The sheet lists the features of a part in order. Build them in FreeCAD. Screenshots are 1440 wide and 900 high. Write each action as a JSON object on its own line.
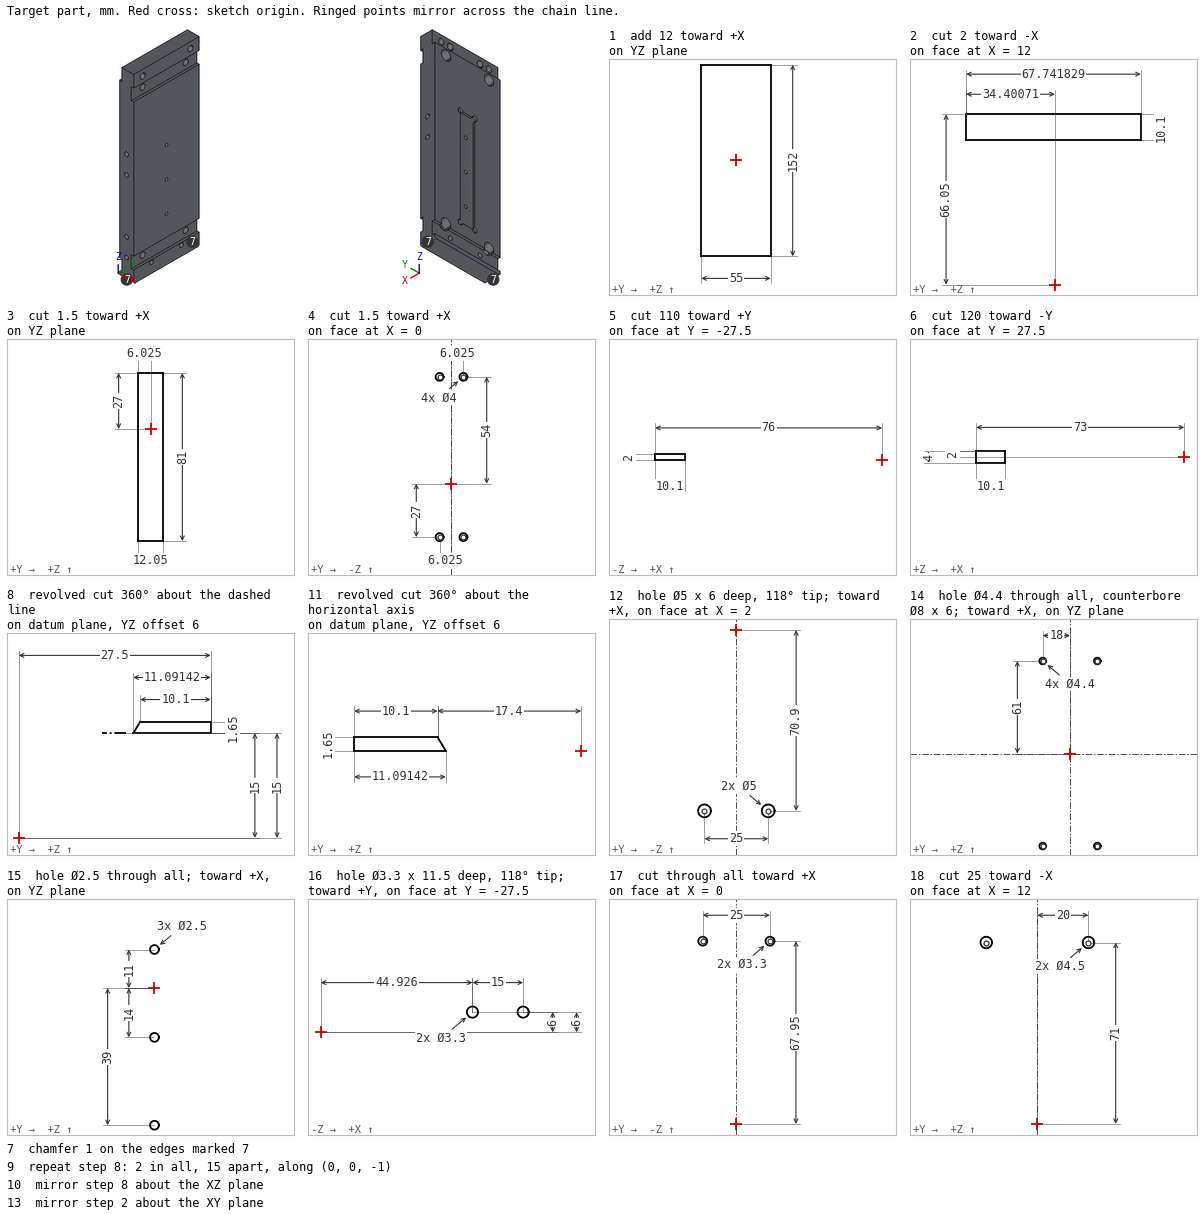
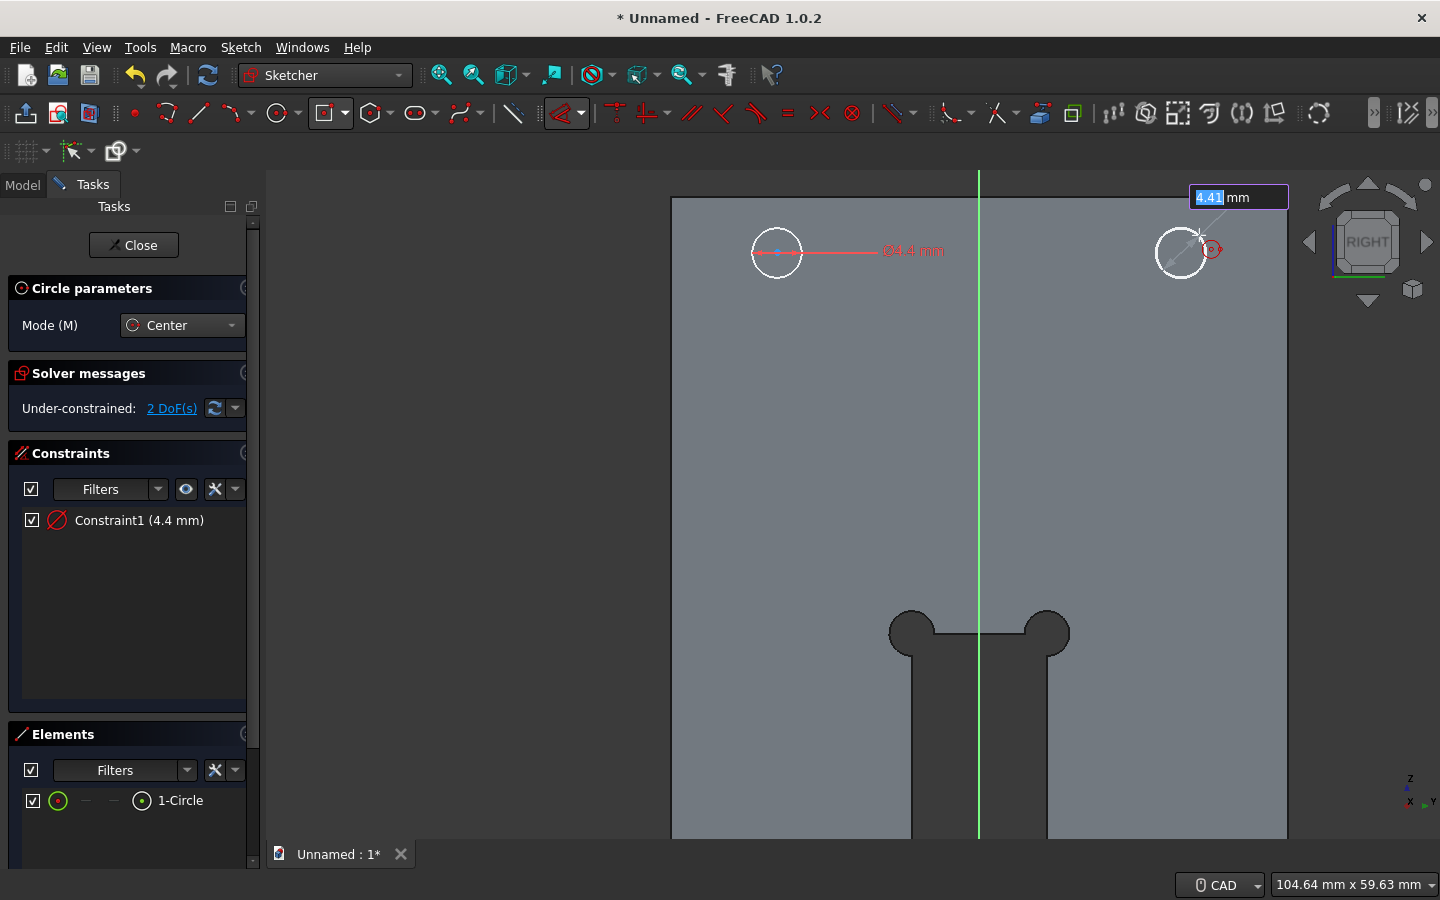
{"action": "type", "text": "4.4"}
{"action": "key", "text": "Return"}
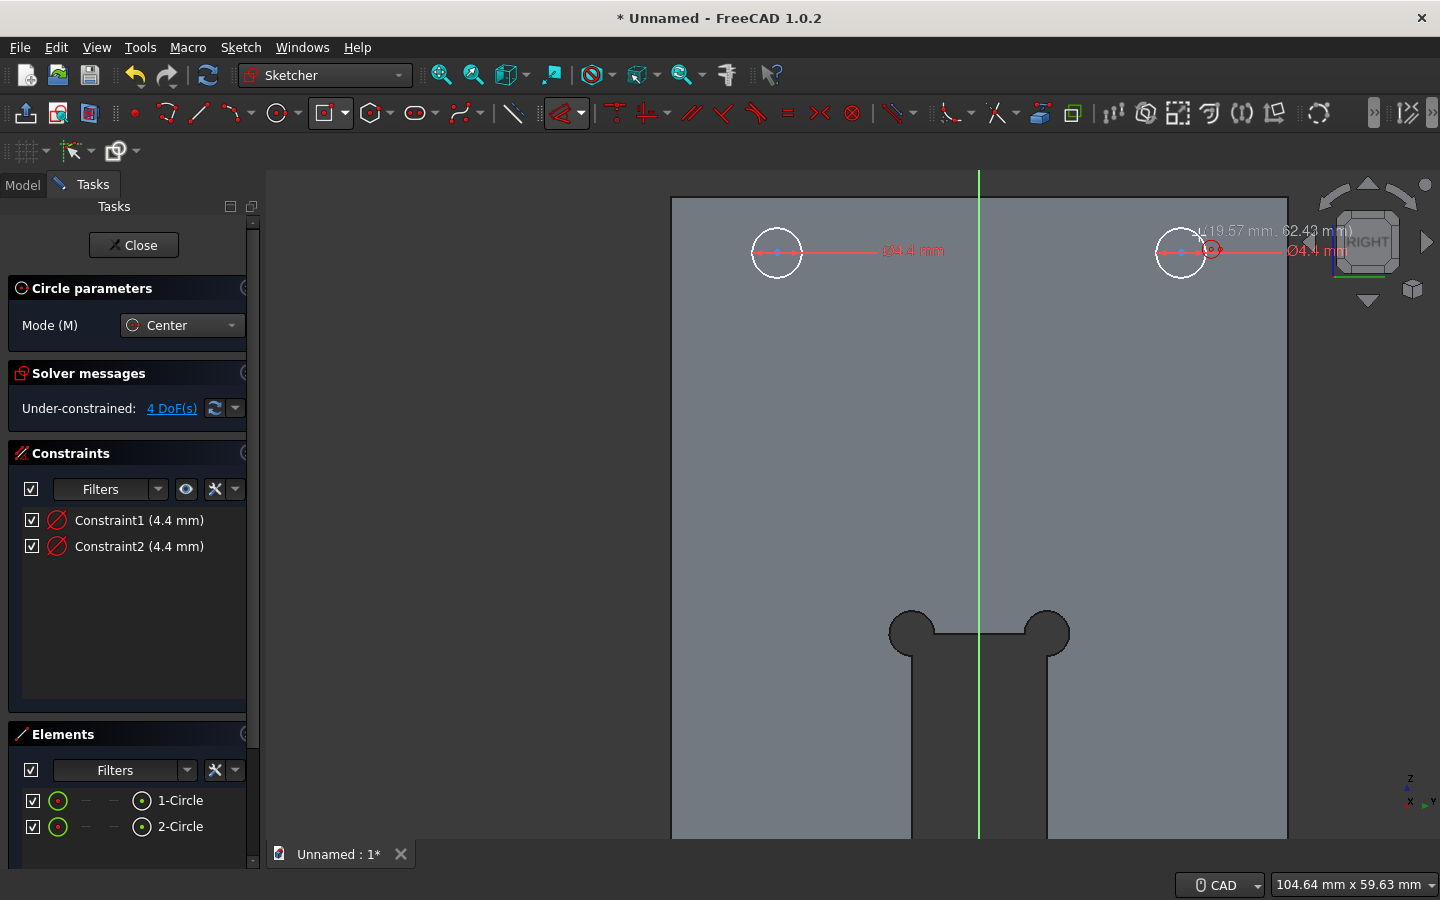
{"action": "scroll", "coordinate": [700, 318], "scroll_direction": "down", "scroll_amount": 6}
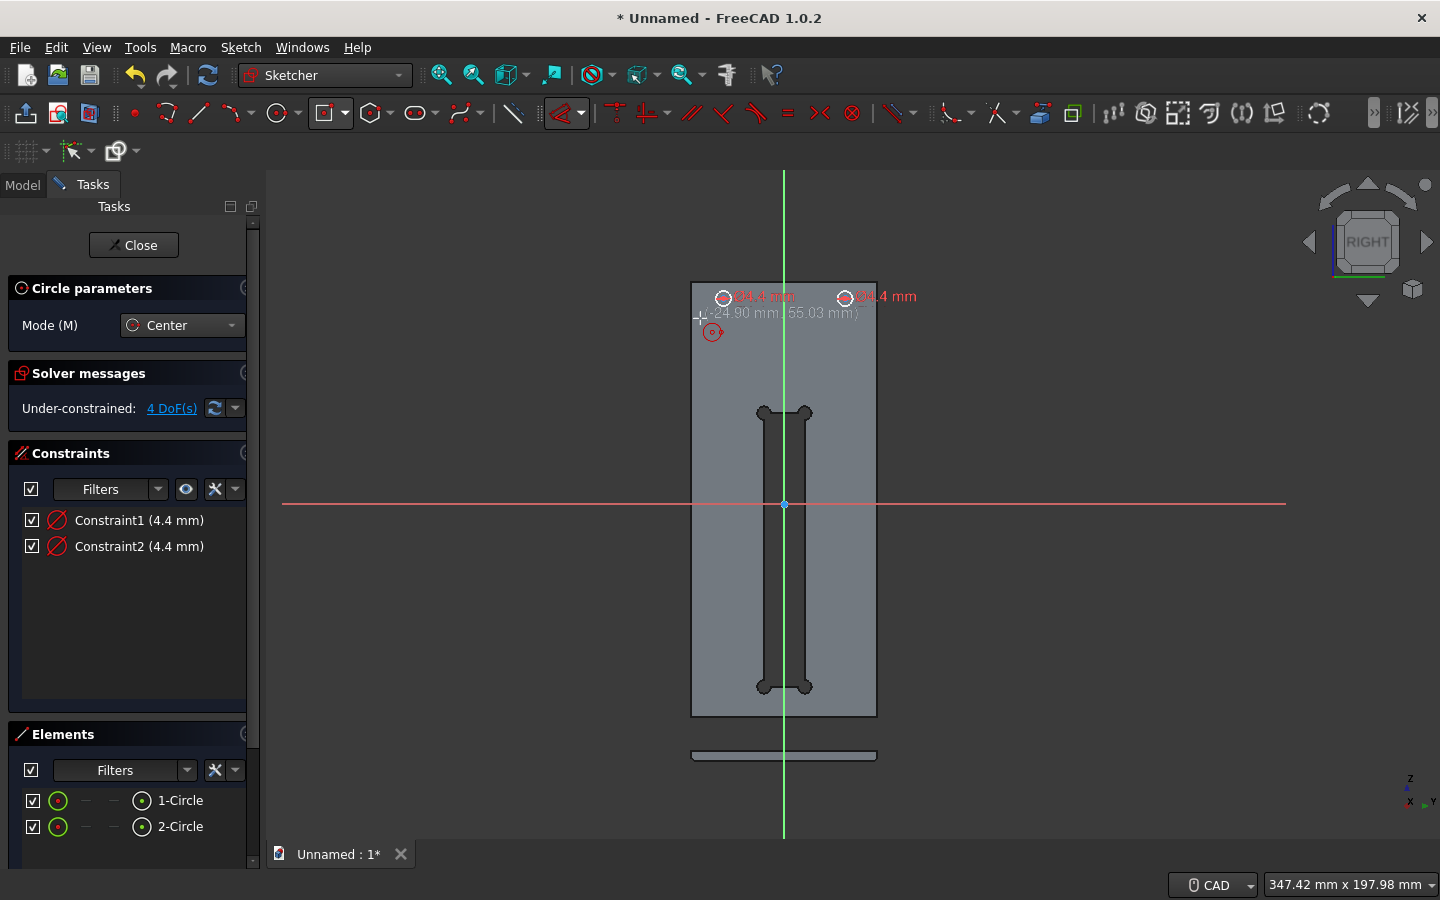
{"action": "scroll", "coordinate": [845, 711], "scroll_direction": "up", "scroll_amount": 6}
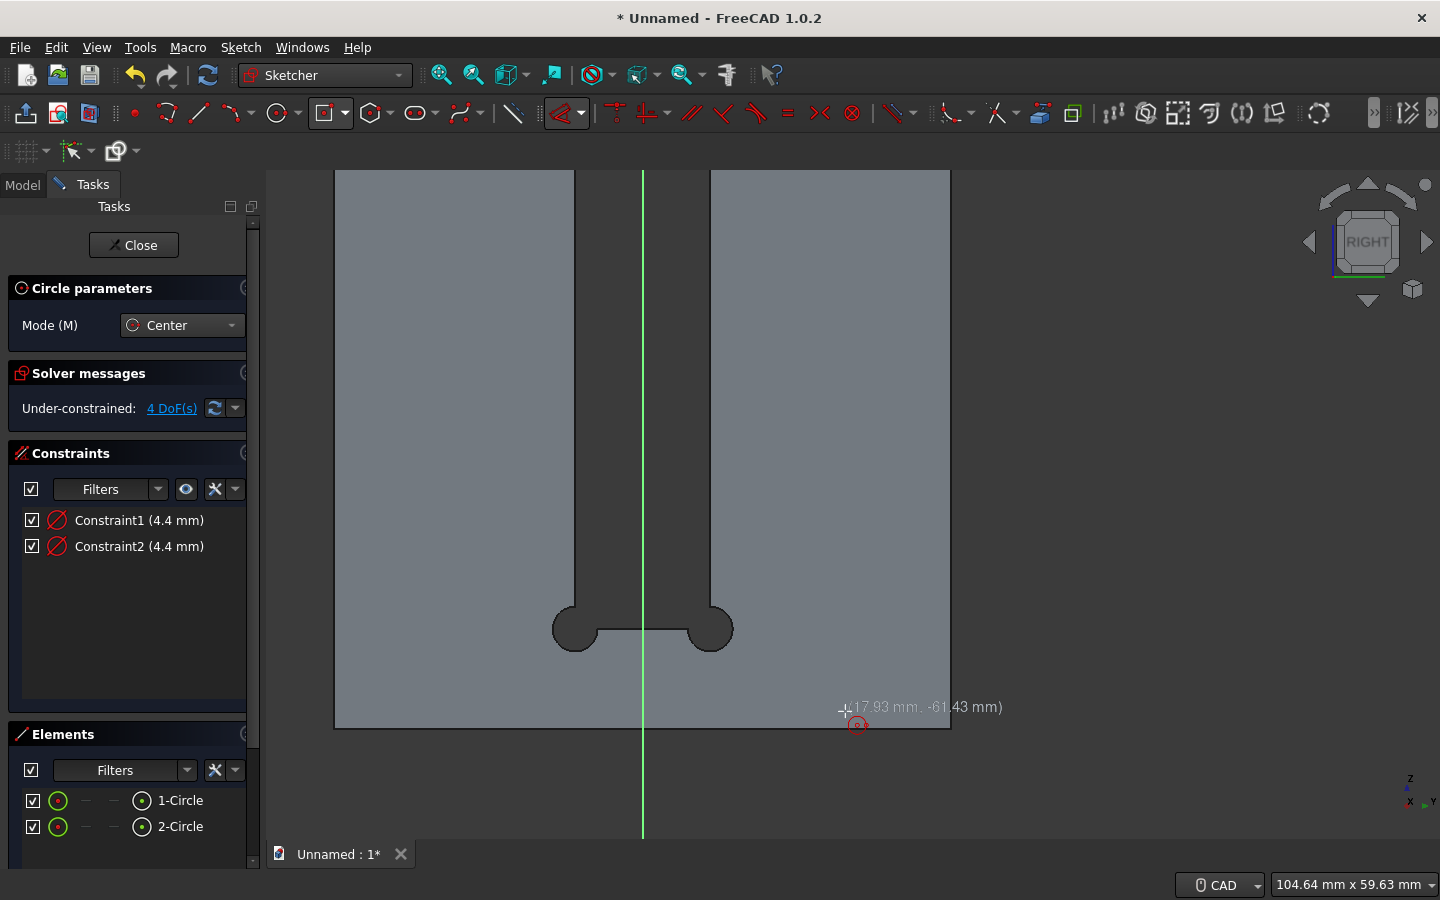
{"action": "left_click", "coordinate": [845, 708]}
{"action": "mouse_move", "coordinate": [862, 690]}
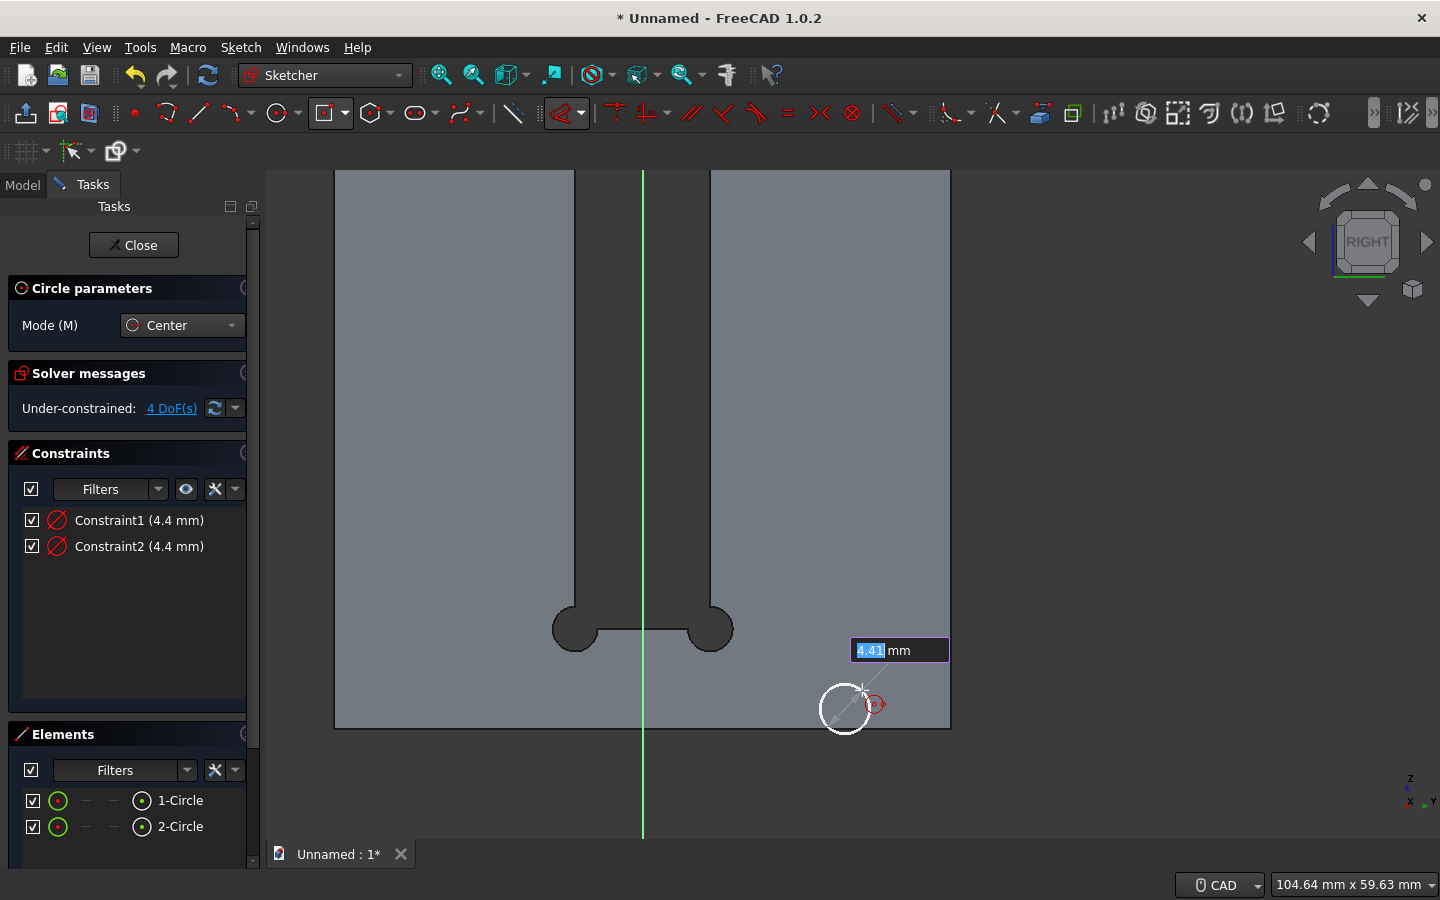
{"action": "type", "text": "4.4"}
{"action": "key", "text": "Return"}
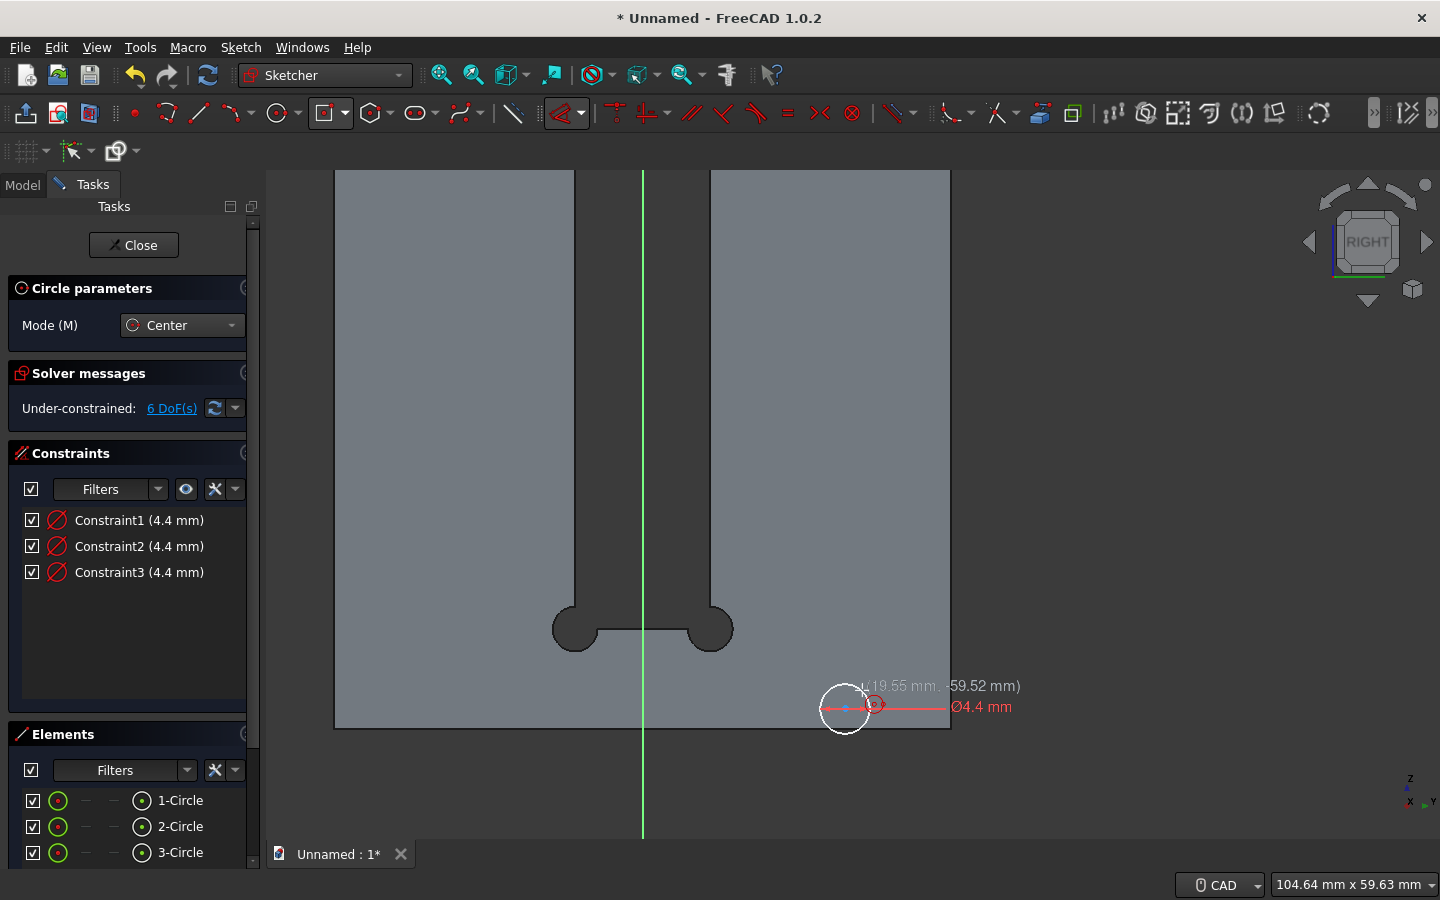
{"action": "left_click", "coordinate": [441, 708]}
{"action": "mouse_move", "coordinate": [458, 690]}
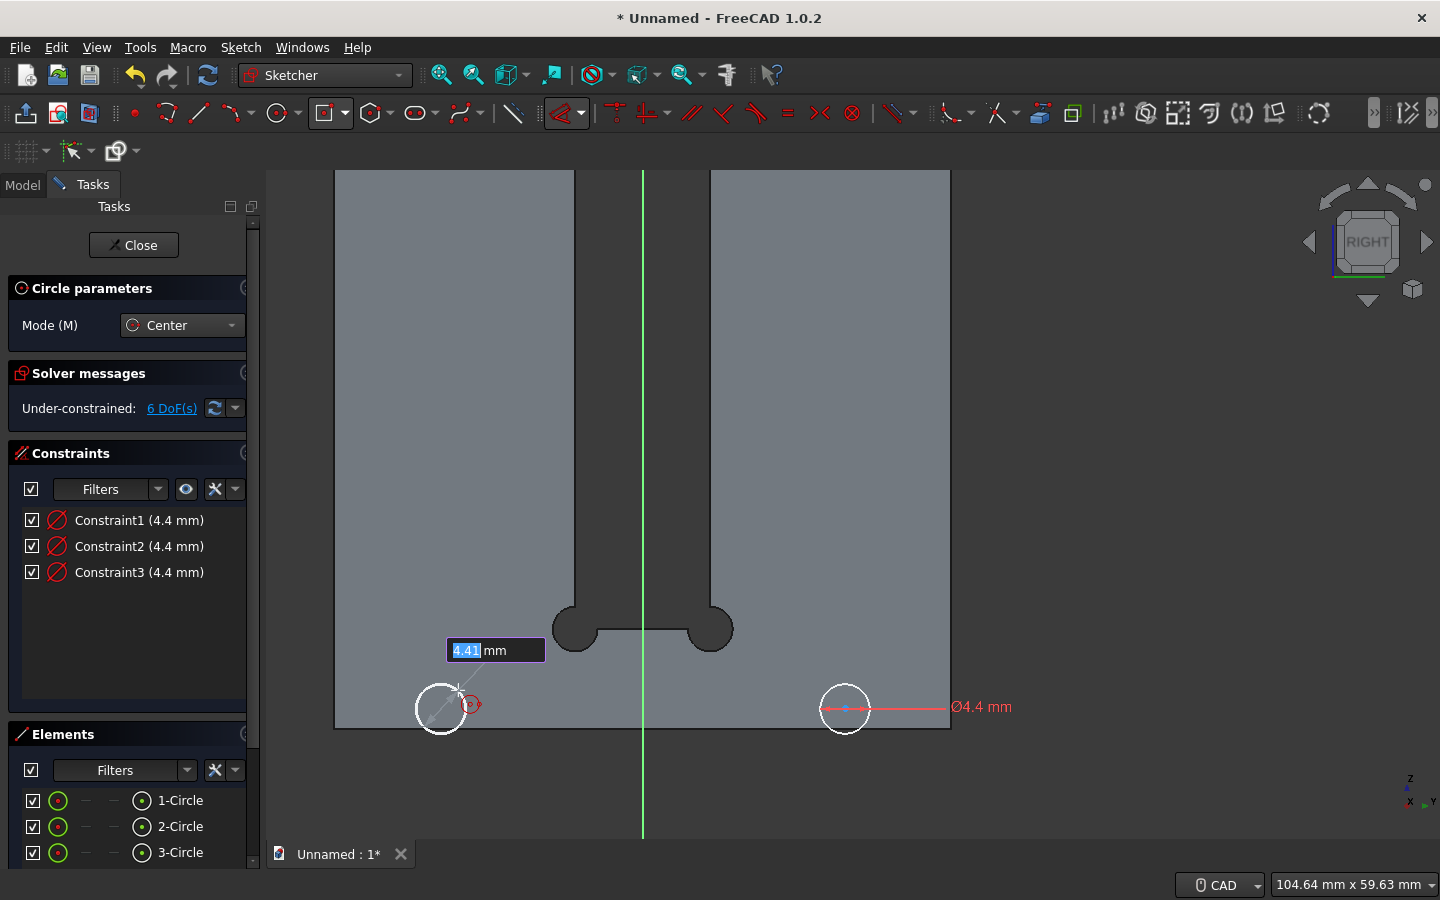
{"action": "type", "text": "4.4"}
{"action": "key", "text": "Return"}
{"action": "key", "text": "Escape"}